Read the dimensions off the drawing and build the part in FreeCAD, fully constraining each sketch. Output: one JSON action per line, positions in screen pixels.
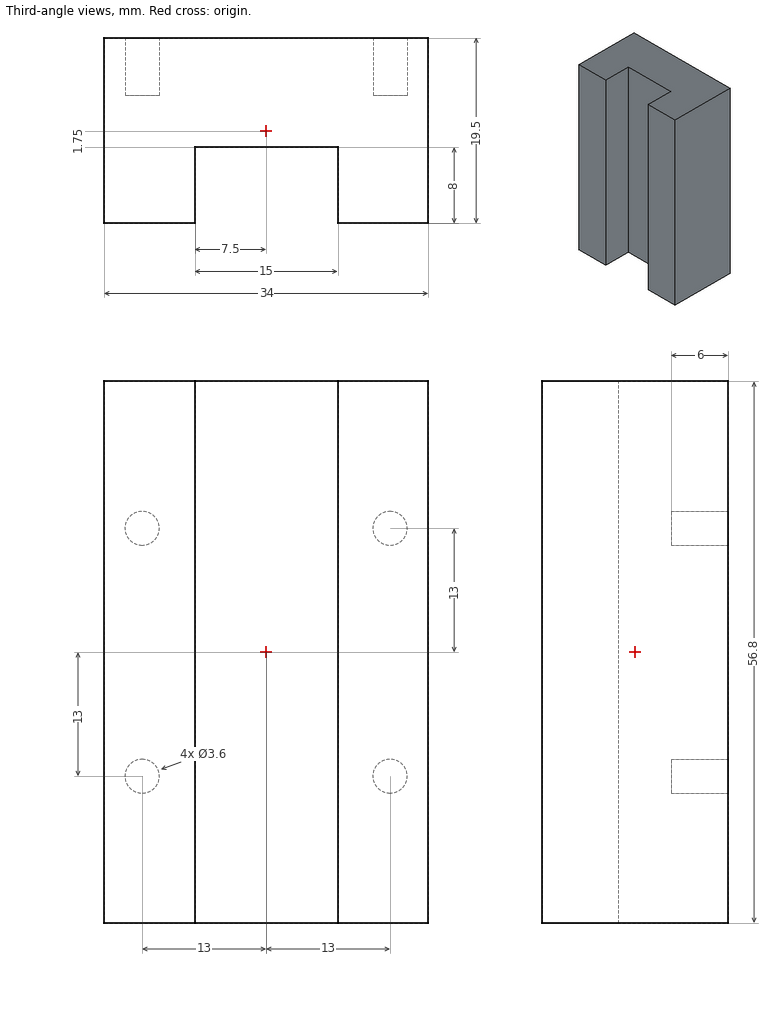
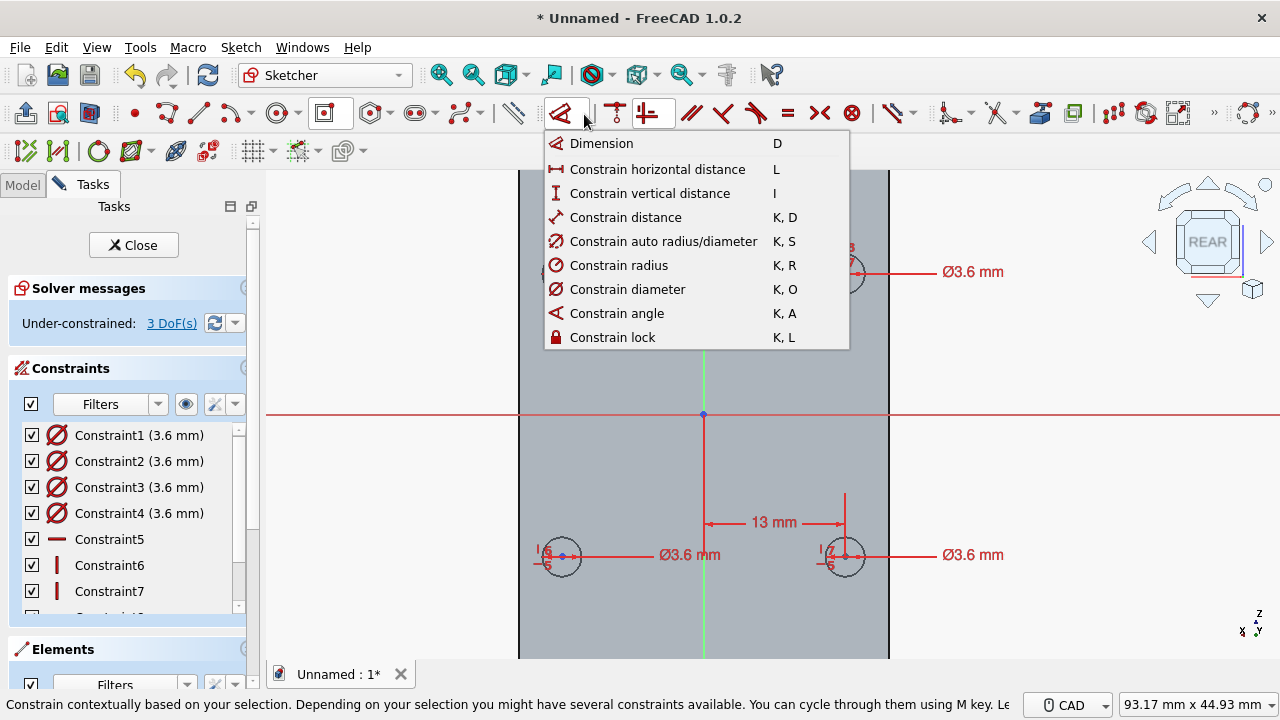
{"action": "left_click", "coordinate": [697, 193]}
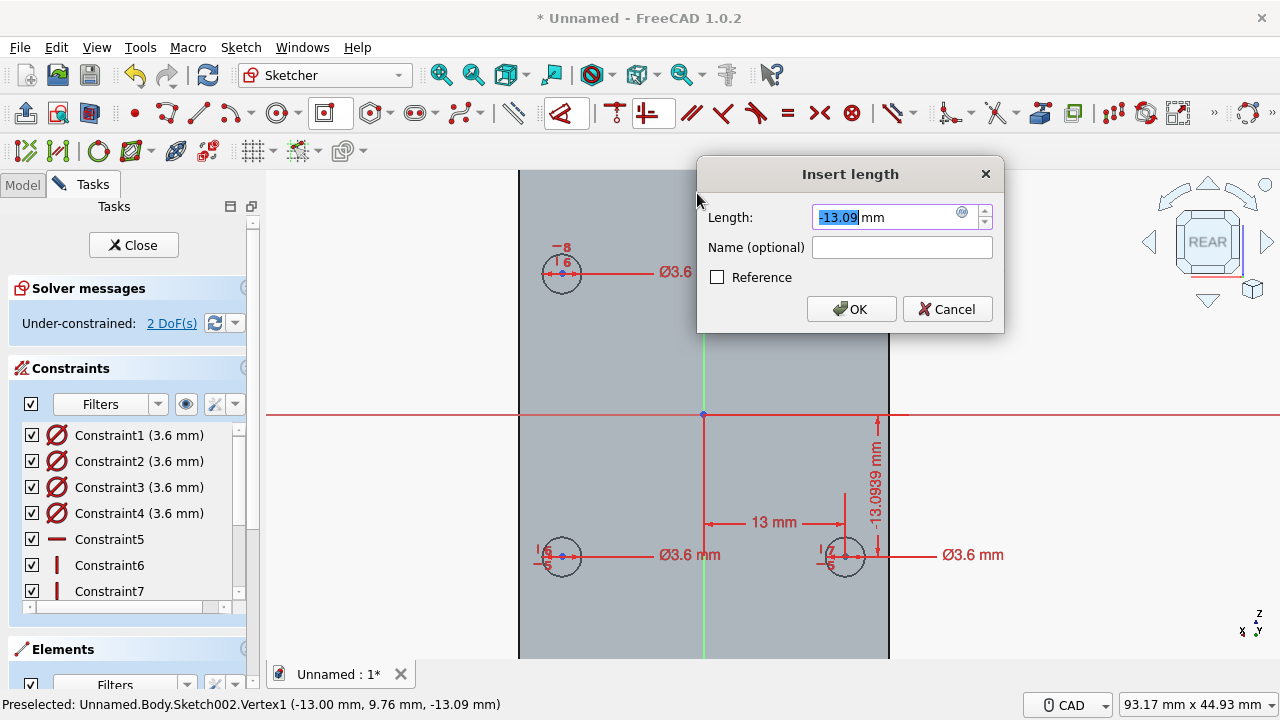
{"action": "type", "text": "-13"}
{"action": "key", "text": "Return"}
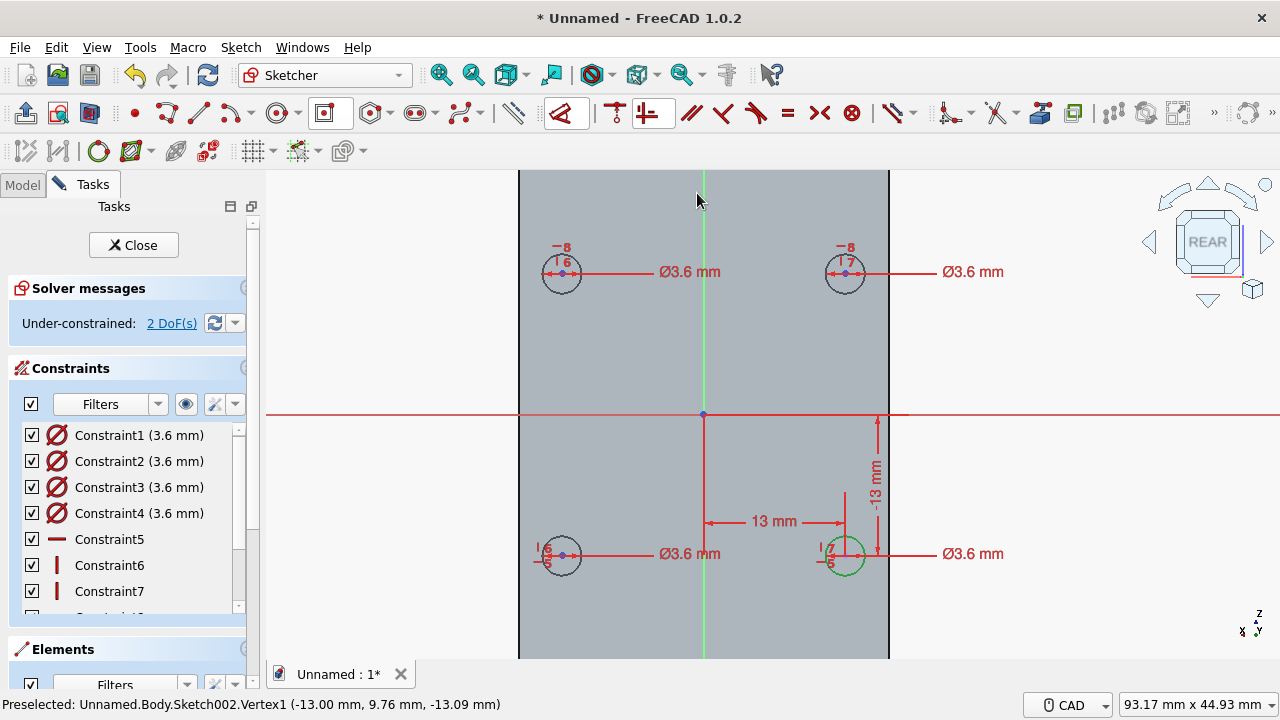
{"action": "left_click", "coordinate": [562, 556]}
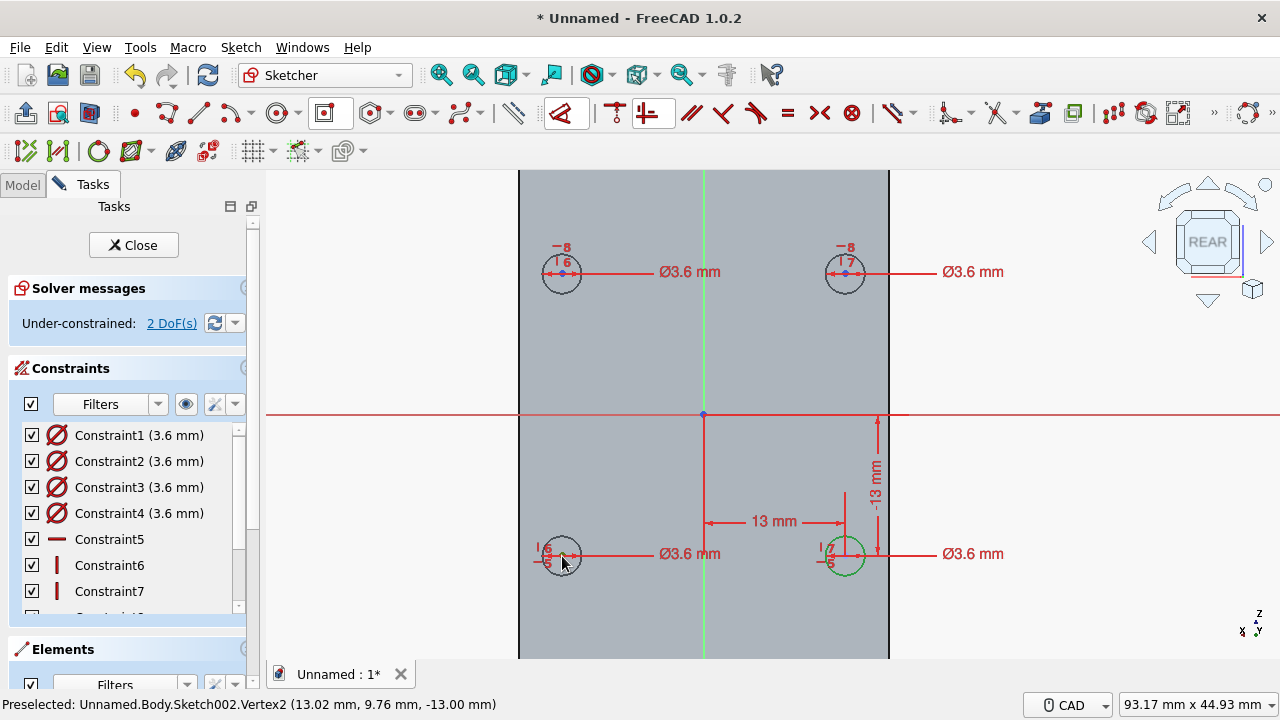
{"action": "left_click", "coordinate": [584, 114]}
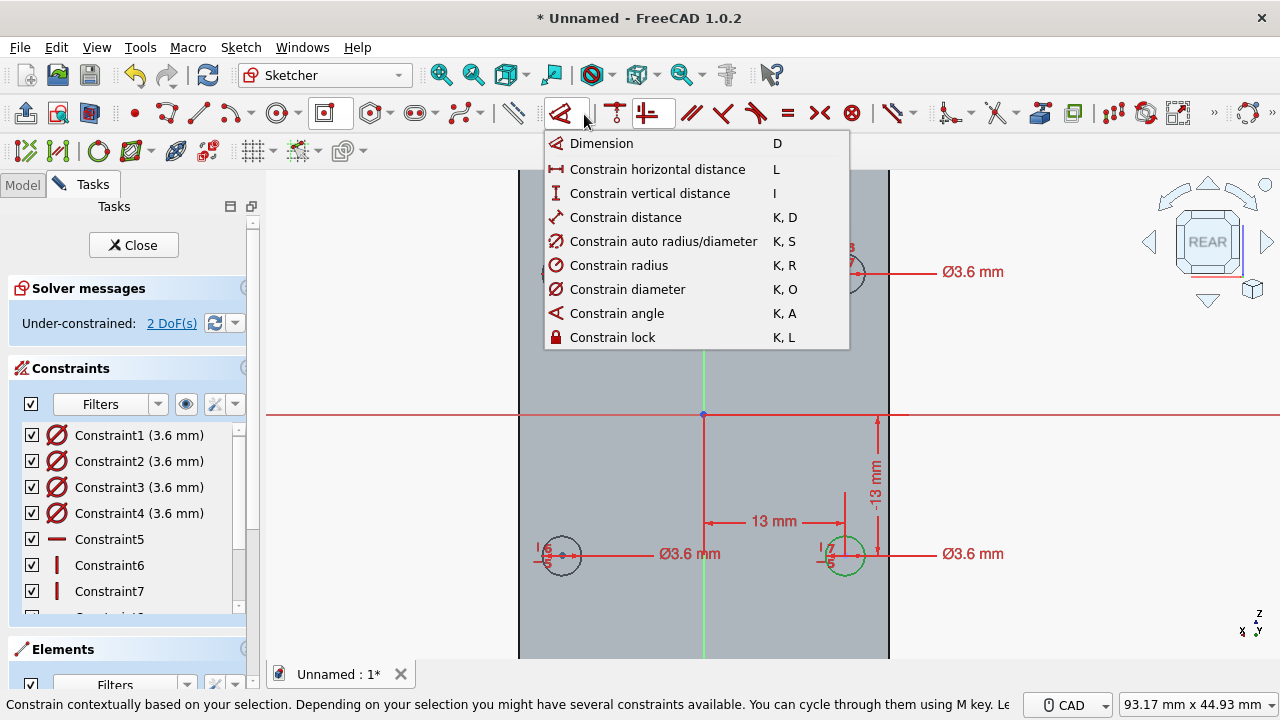
{"action": "left_click", "coordinate": [697, 169]}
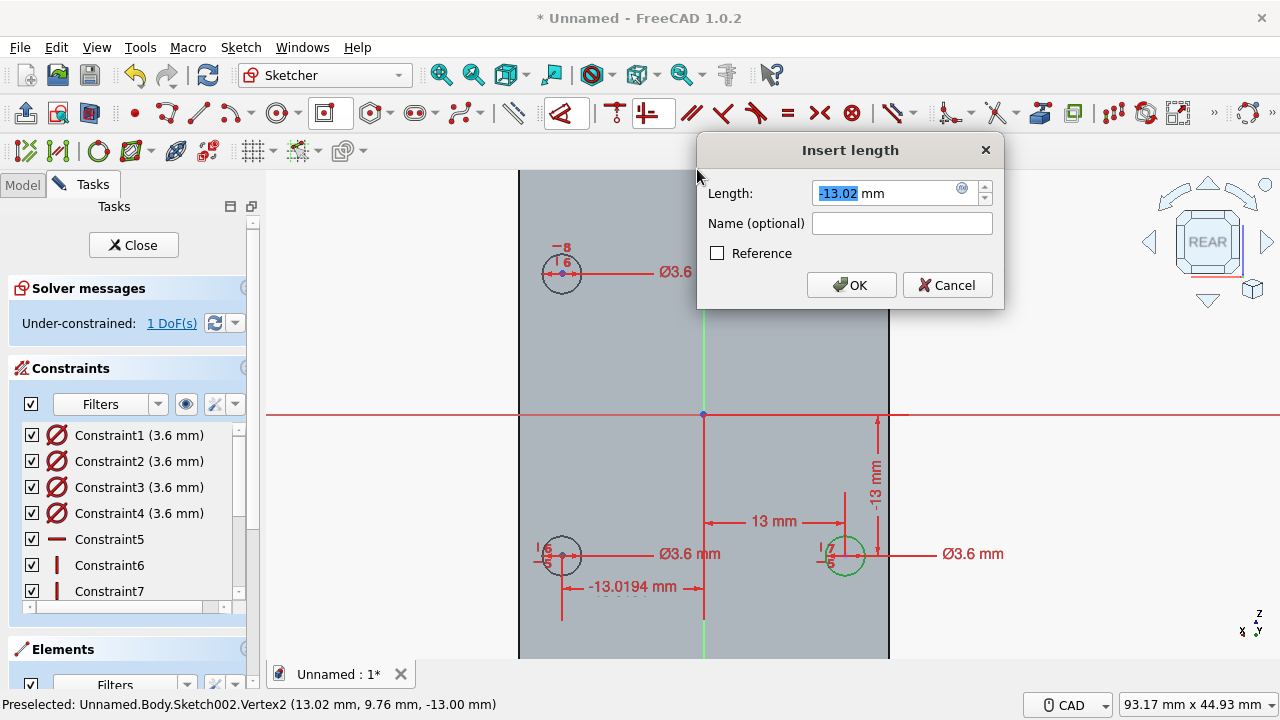
{"action": "type", "text": "-13"}
{"action": "key", "text": "Return"}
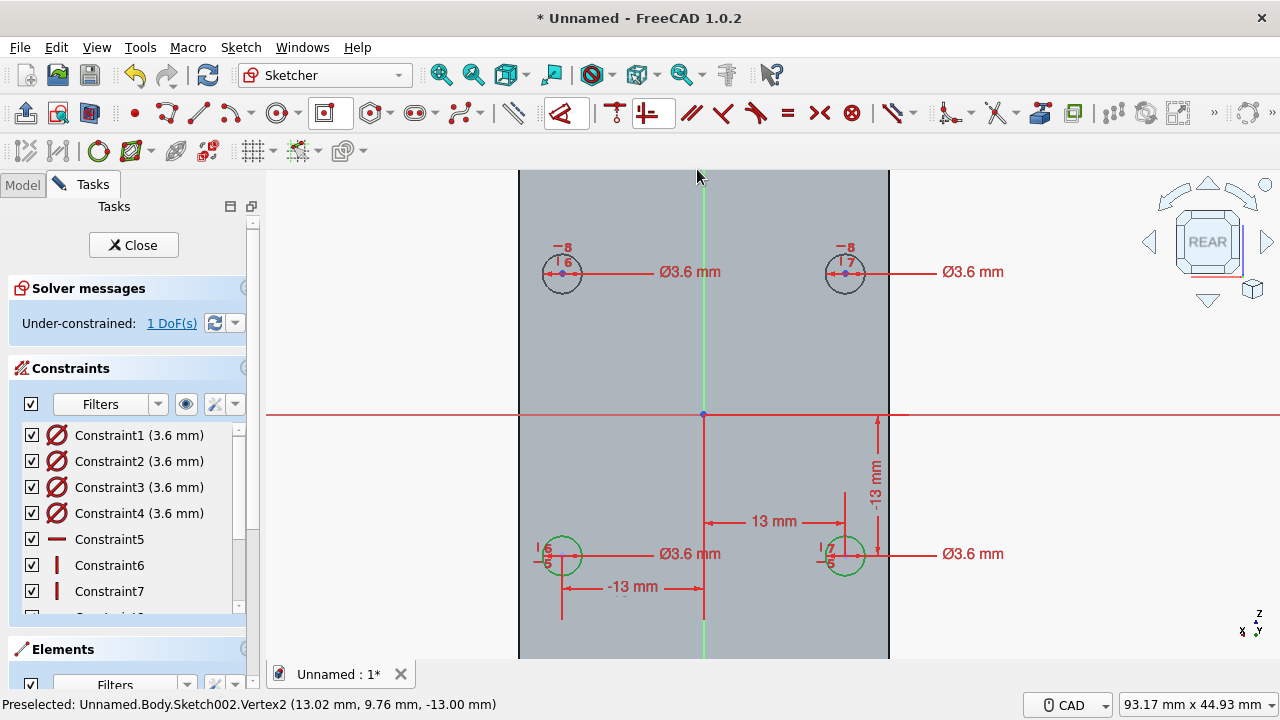
{"action": "left_click", "coordinate": [562, 274]}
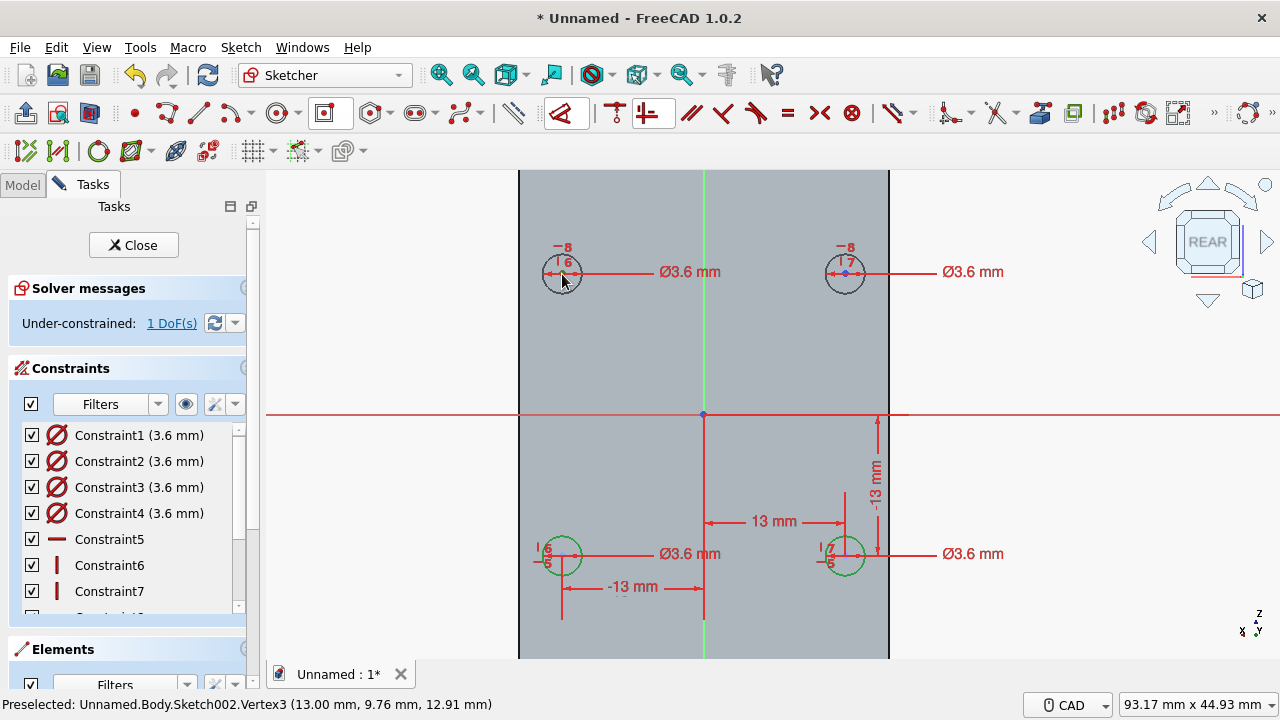
{"action": "left_click", "coordinate": [584, 114]}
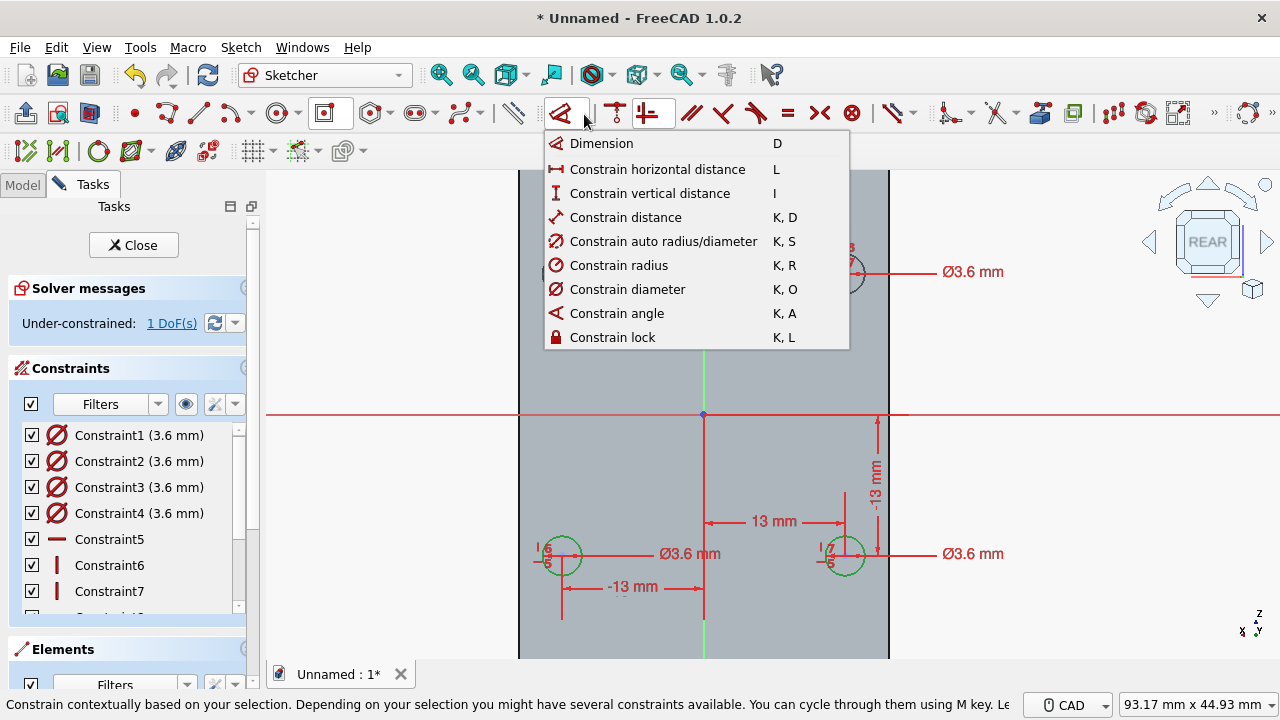
{"action": "left_click", "coordinate": [697, 193]}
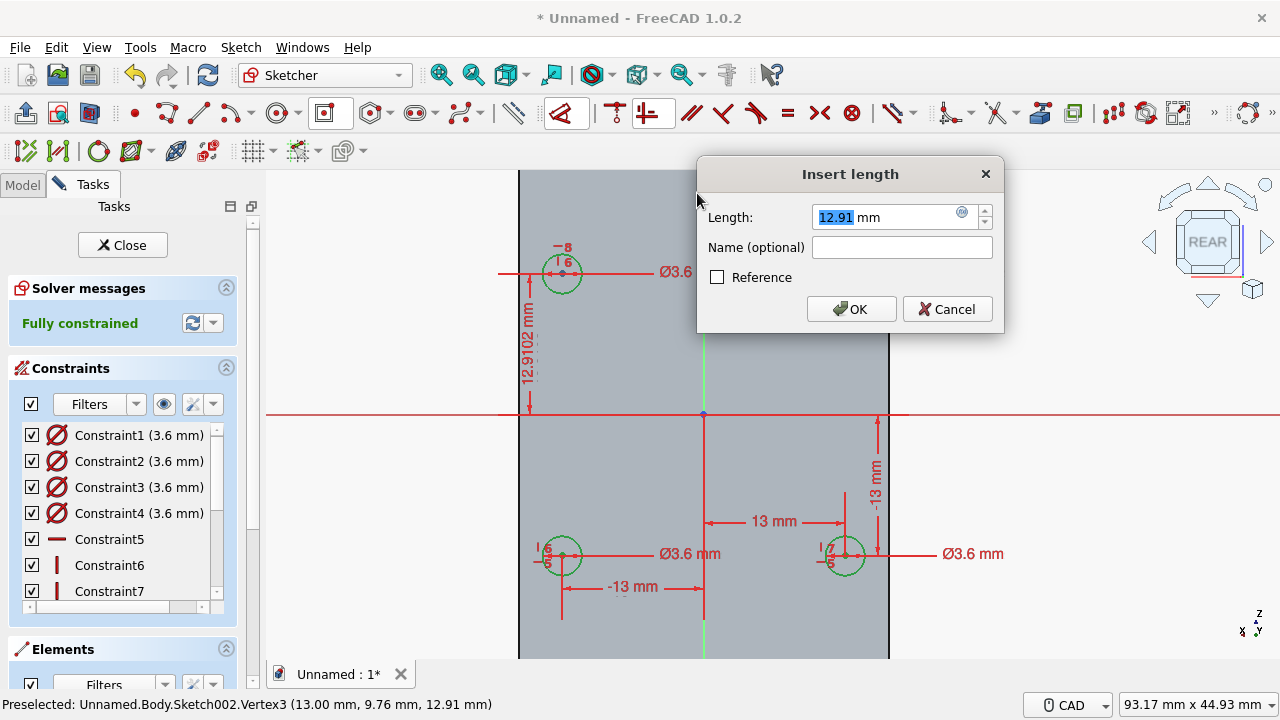
{"action": "type", "text": "13"}
{"action": "key", "text": "Return"}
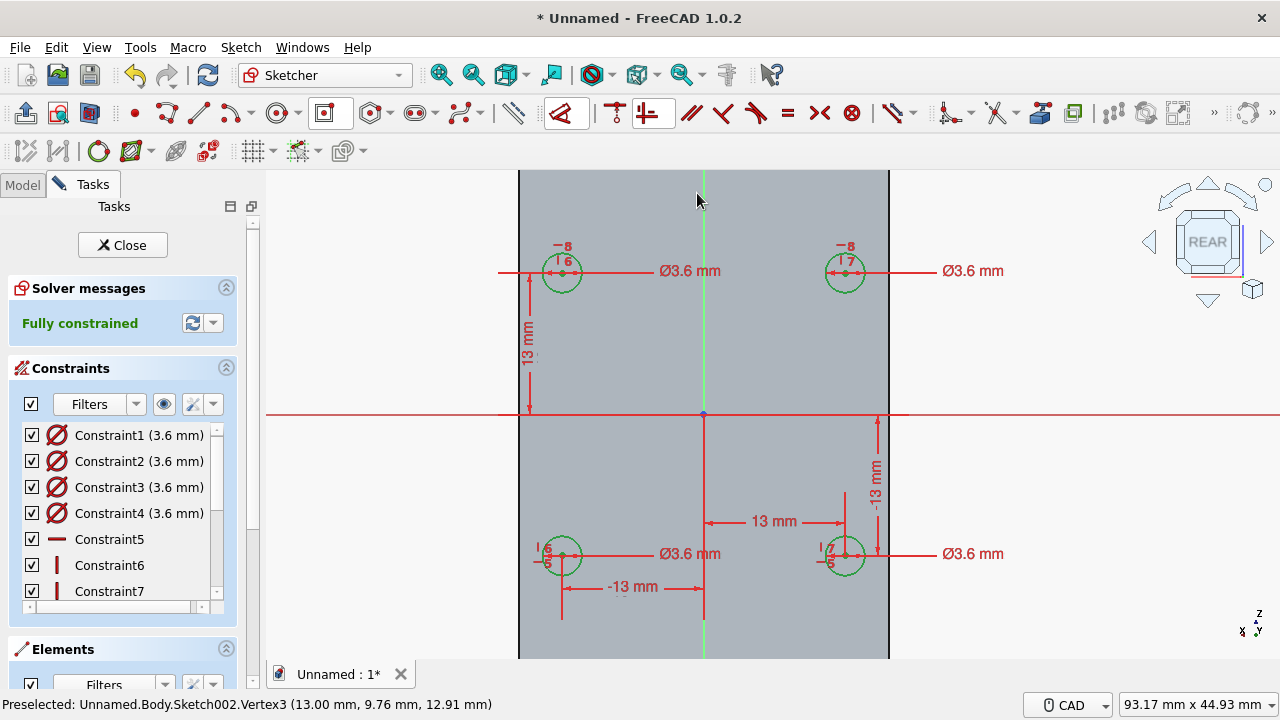
{"action": "left_click", "coordinate": [123, 245]}